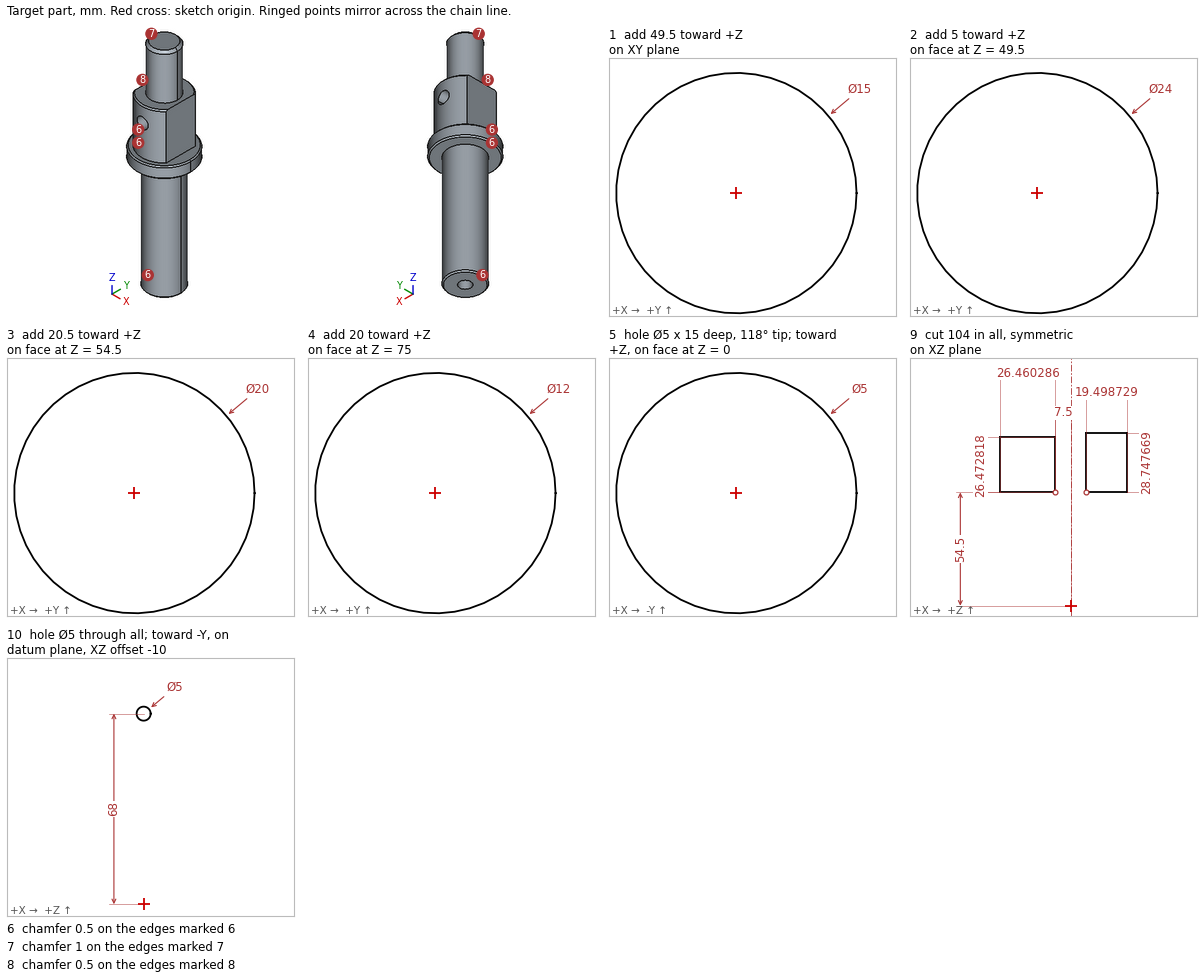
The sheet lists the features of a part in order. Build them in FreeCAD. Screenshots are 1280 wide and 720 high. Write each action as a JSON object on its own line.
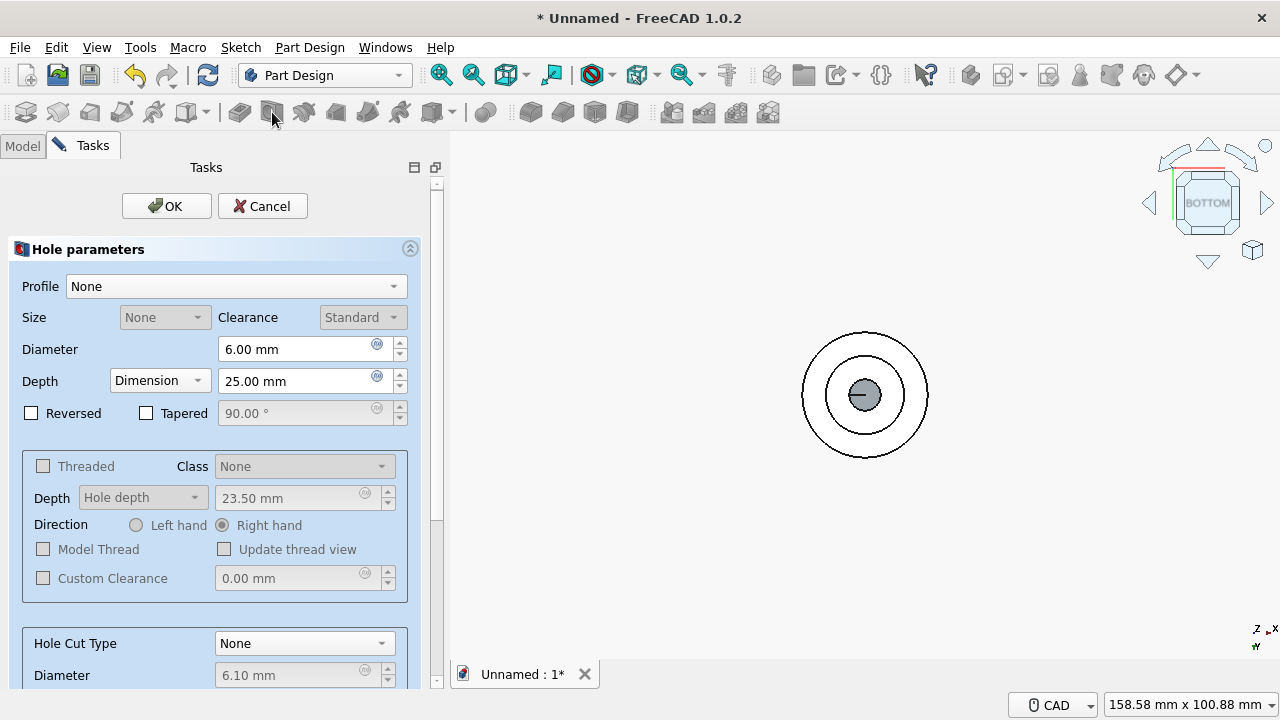
{"action": "triple_click", "coordinate": [305, 349]}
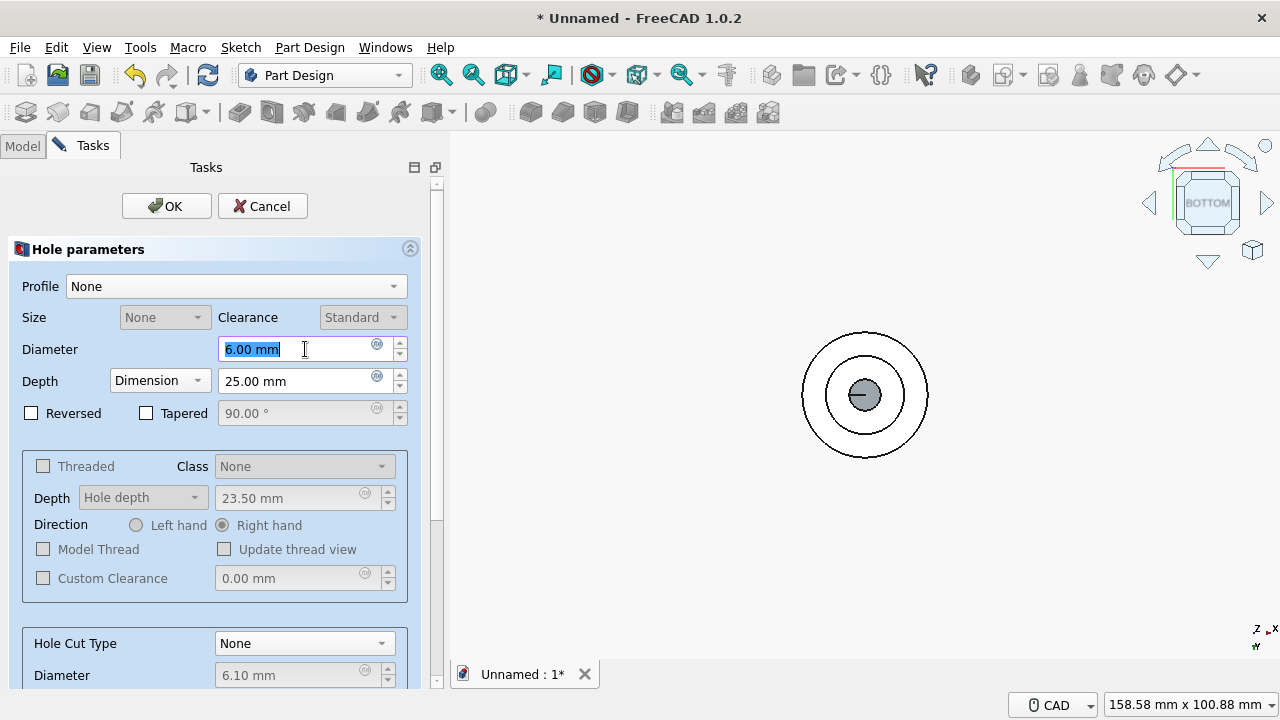
{"action": "type", "text": "5"}
{"action": "key", "text": "Tab"}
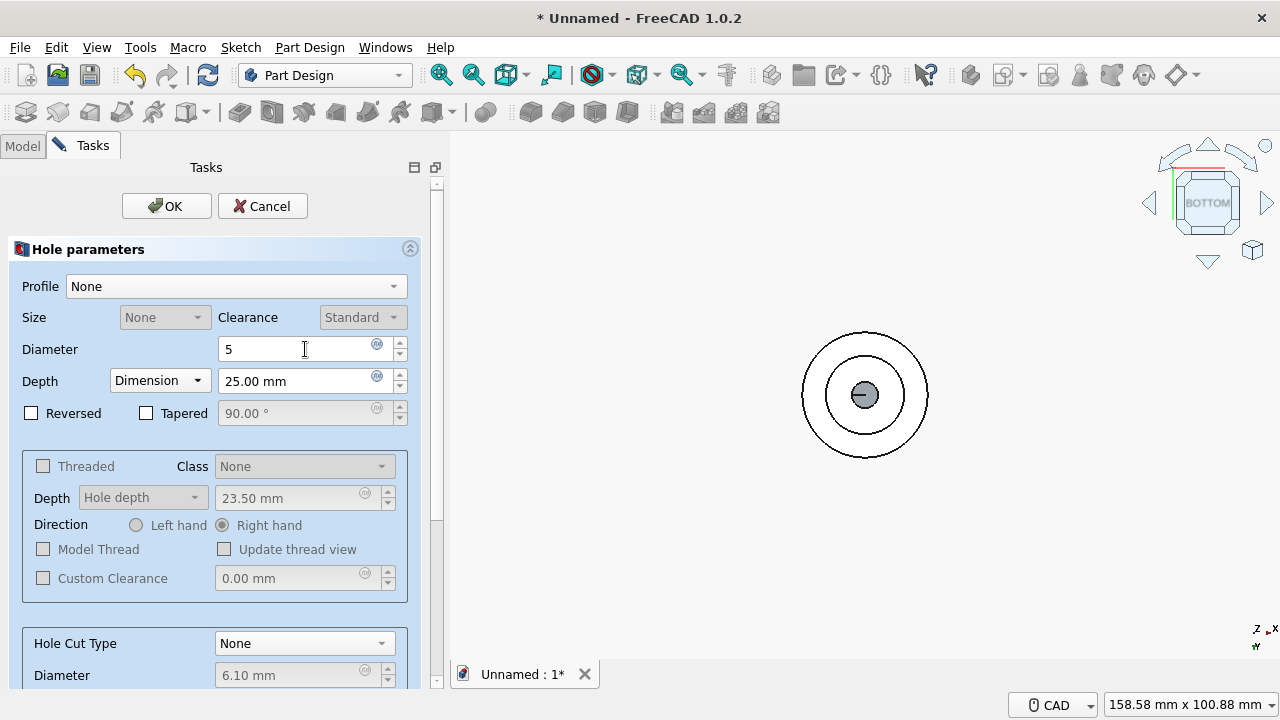
{"action": "triple_click", "coordinate": [305, 381]}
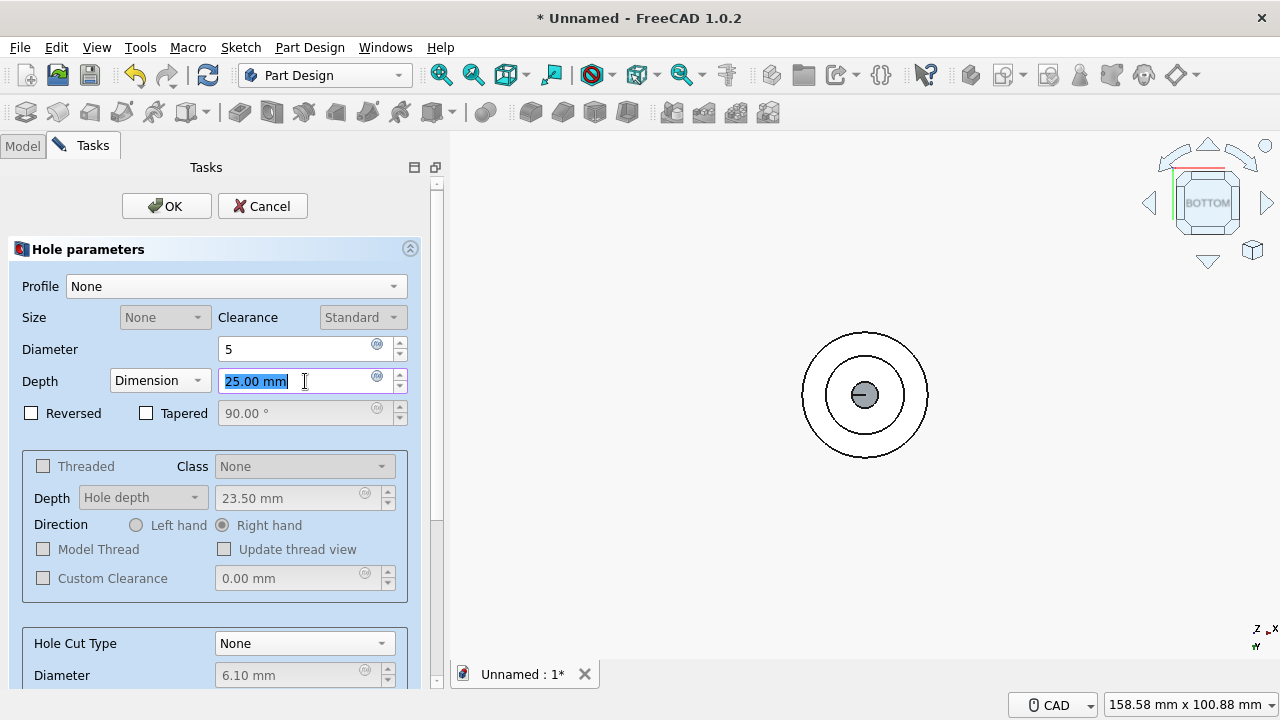
{"action": "type", "text": "15"}
{"action": "key", "text": "Tab"}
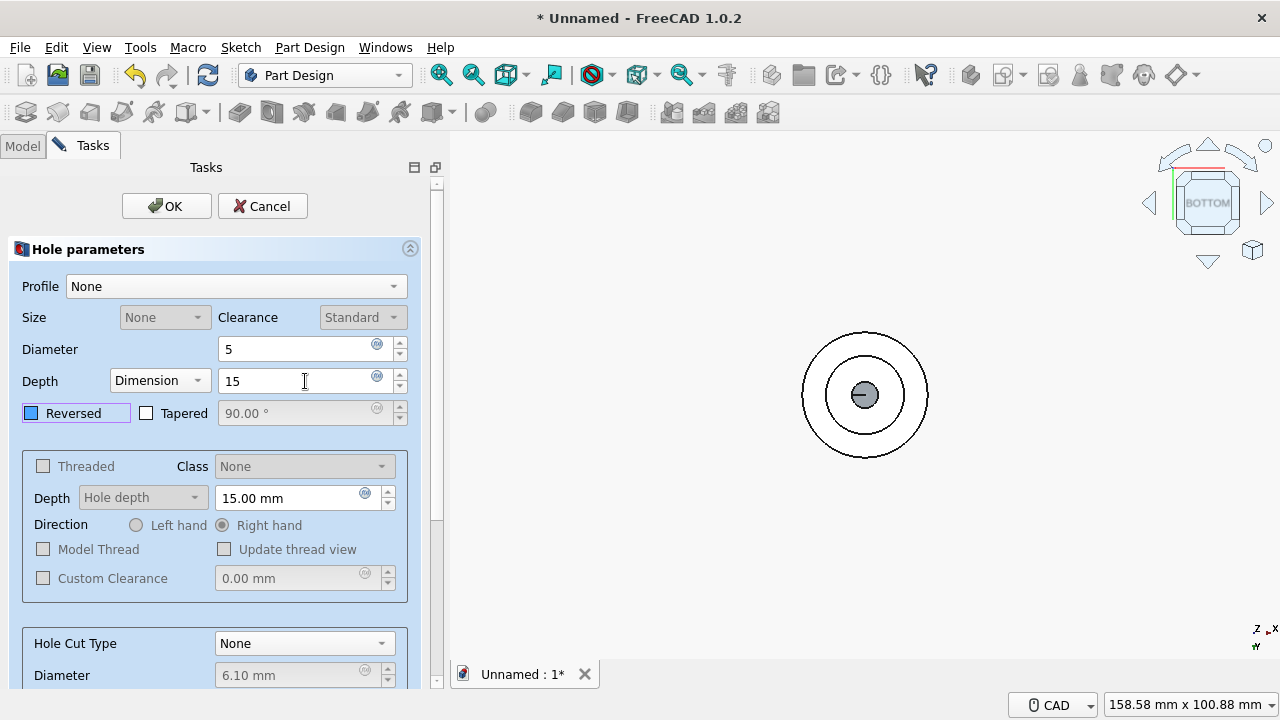
{"action": "left_click", "coordinate": [167, 206]}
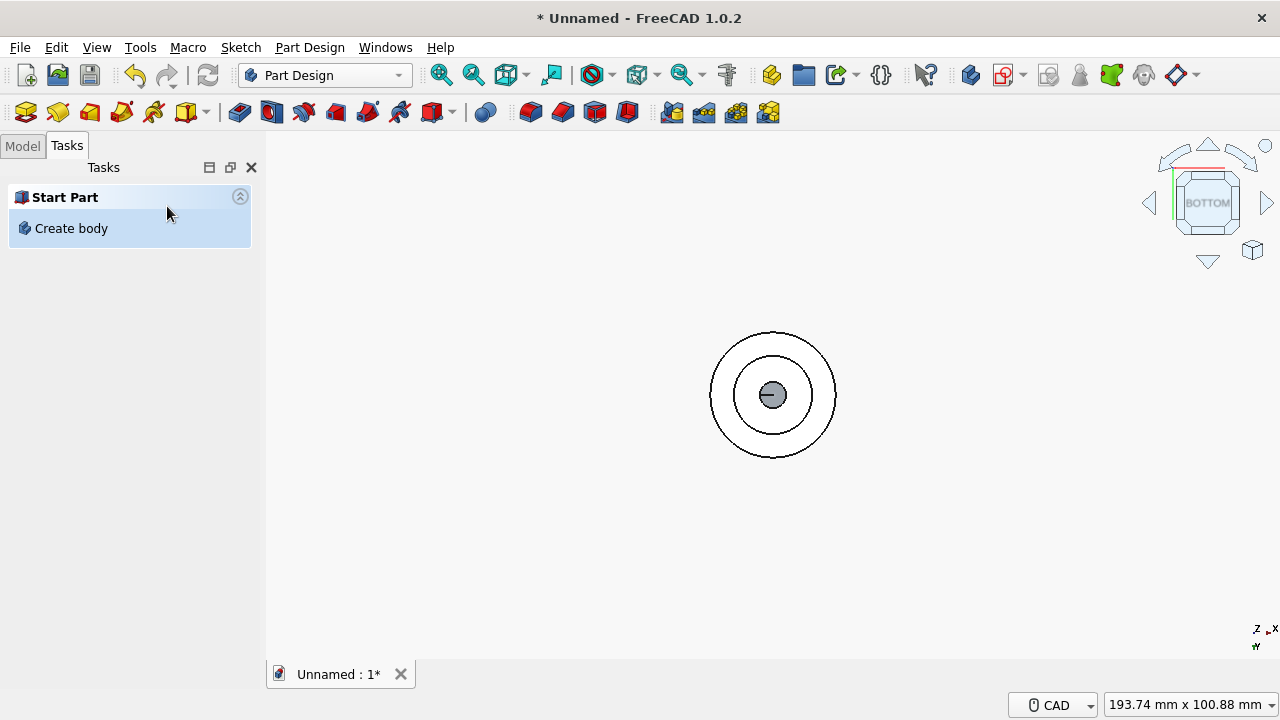
{"action": "key", "text": "v f"}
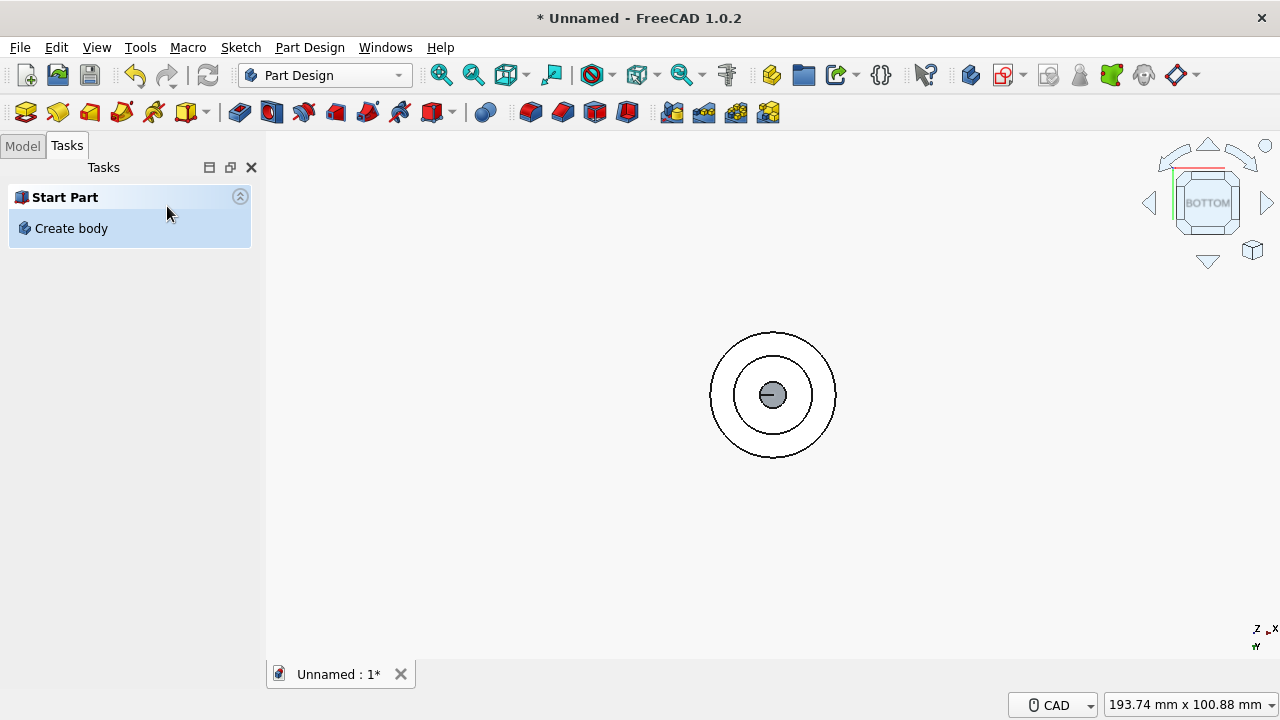
{"action": "left_click", "coordinate": [734, 394]}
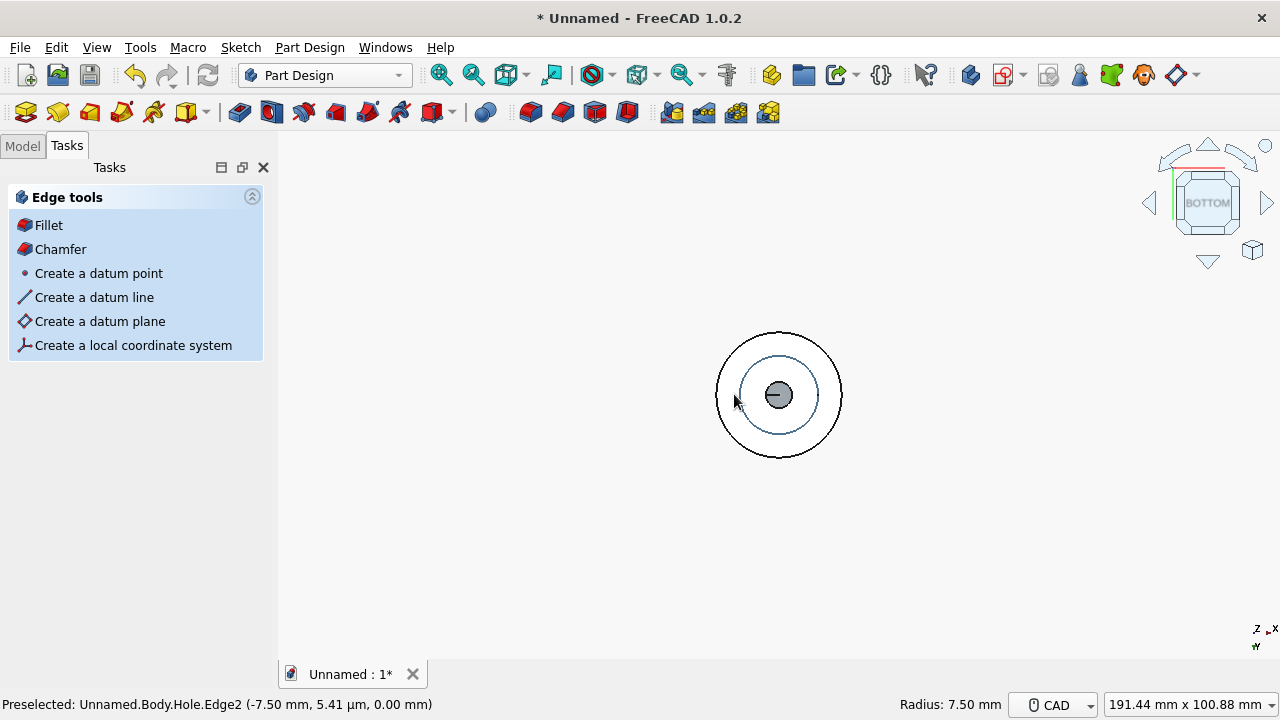
{"action": "left_click", "coordinate": [716, 394], "text": "ctrl"}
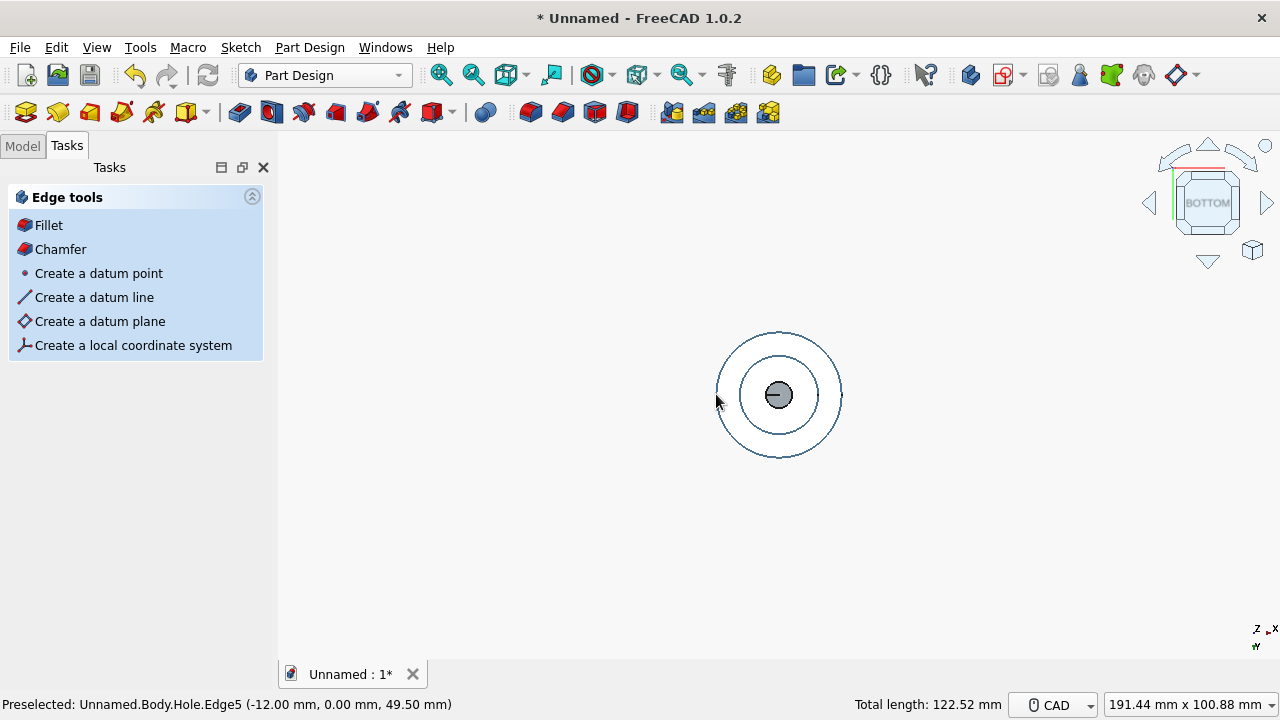
{"action": "key", "text": "0"}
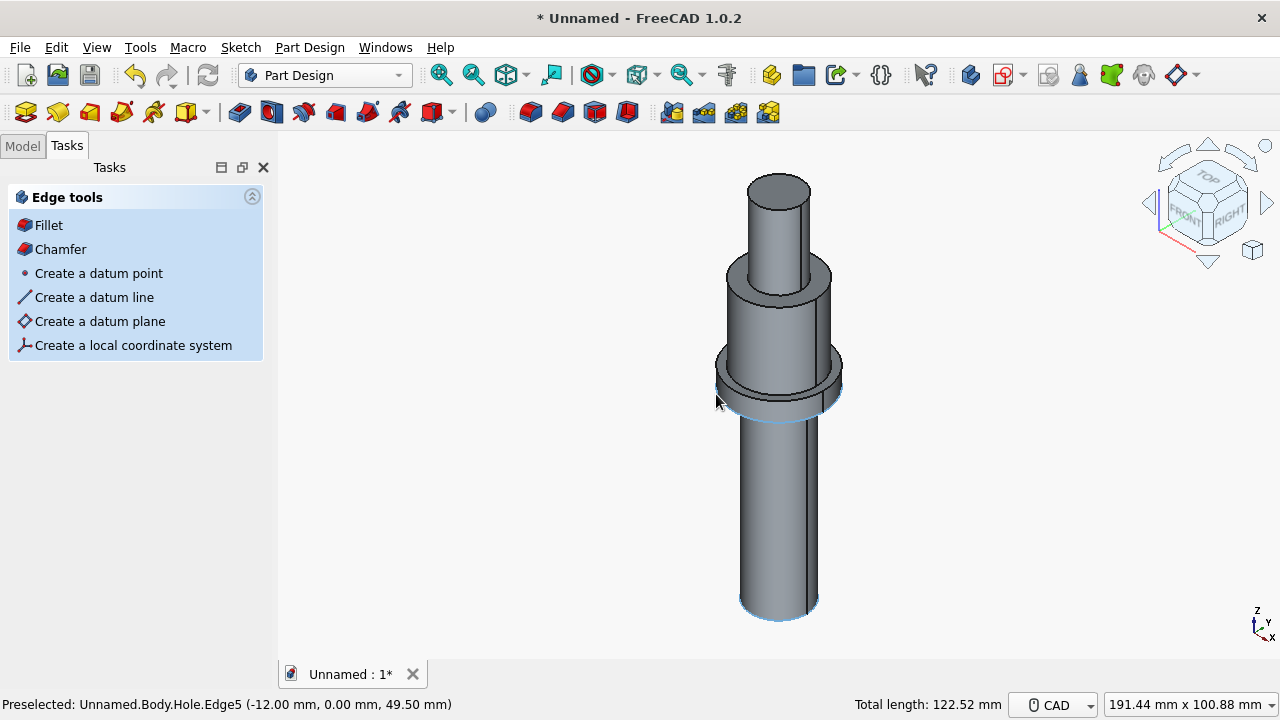
{"action": "left_click", "coordinate": [723, 381], "text": "ctrl"}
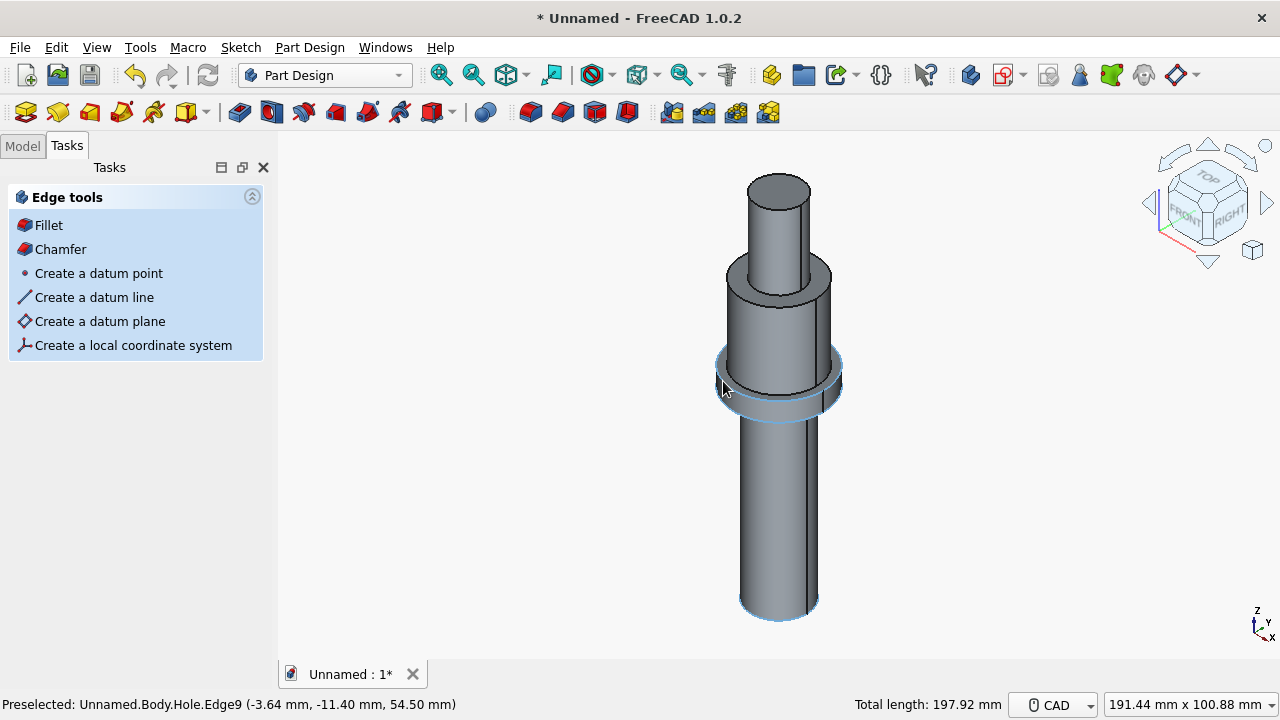
{"action": "left_click", "coordinate": [564, 112]}